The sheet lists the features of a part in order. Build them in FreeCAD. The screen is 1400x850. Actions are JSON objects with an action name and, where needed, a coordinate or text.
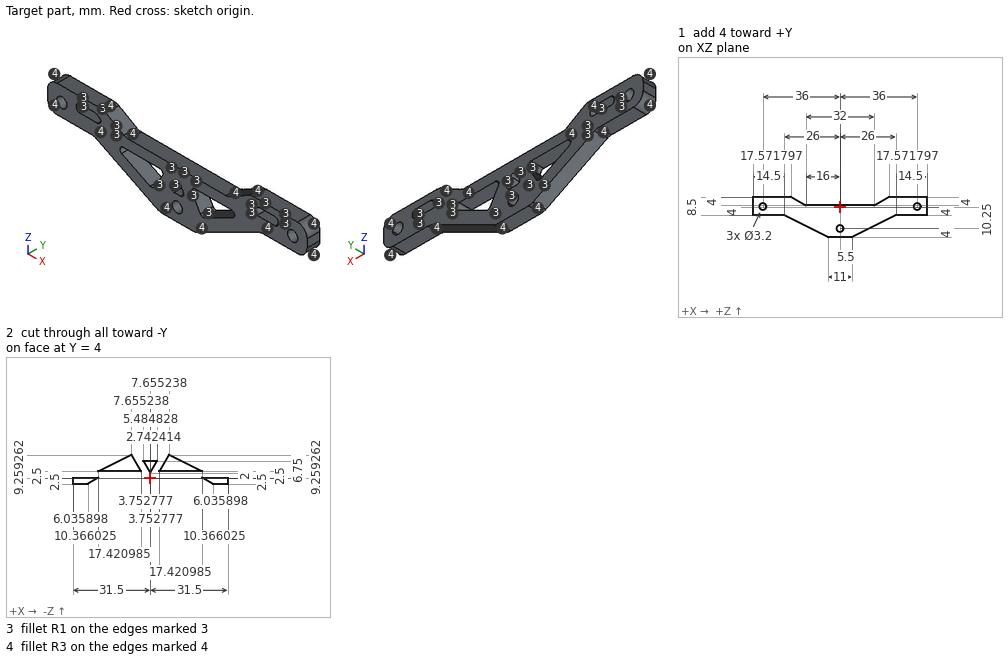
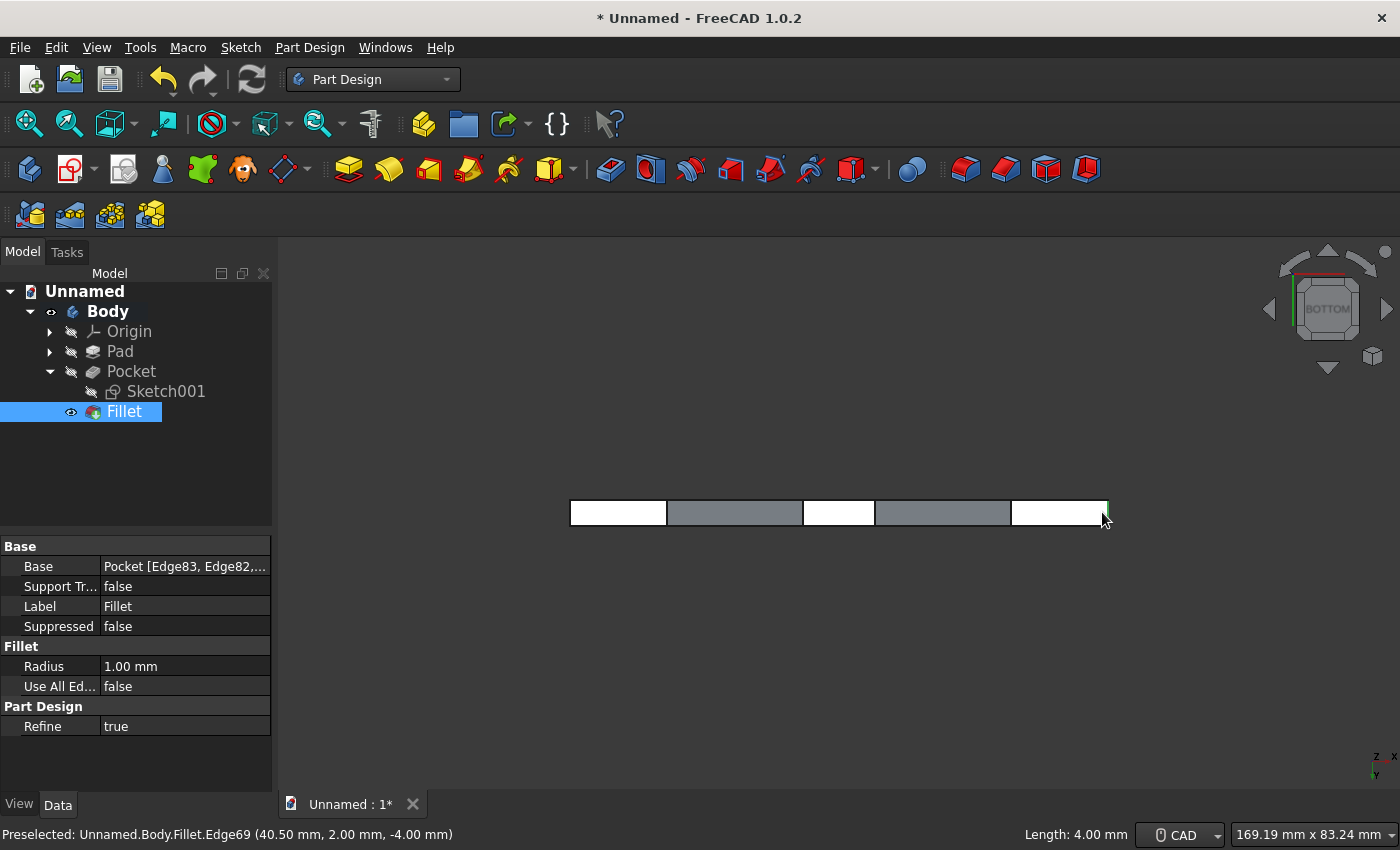
{"action": "left_click", "coordinate": [570, 512], "text": "ctrl"}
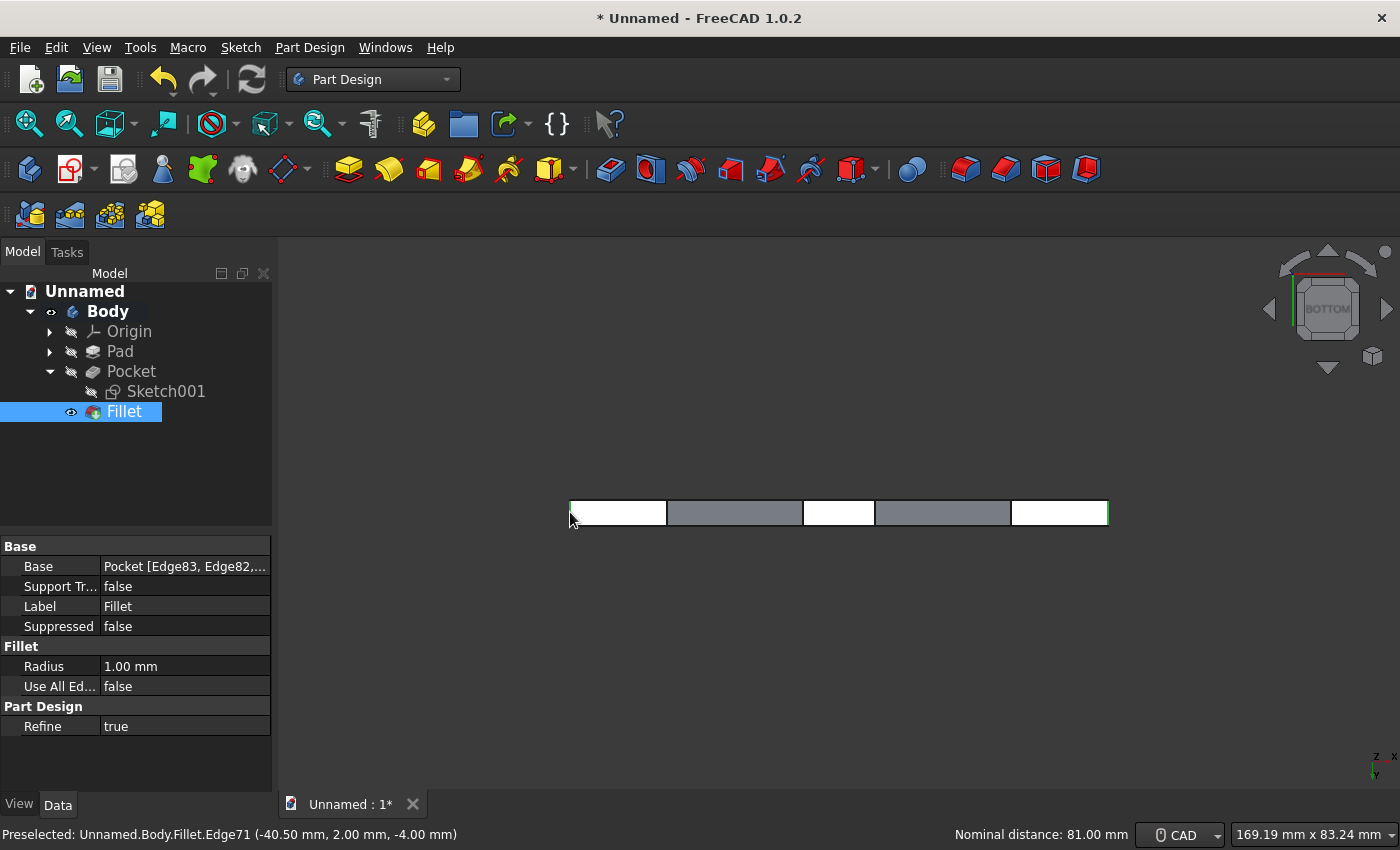
{"action": "left_click", "coordinate": [803, 512], "text": "ctrl"}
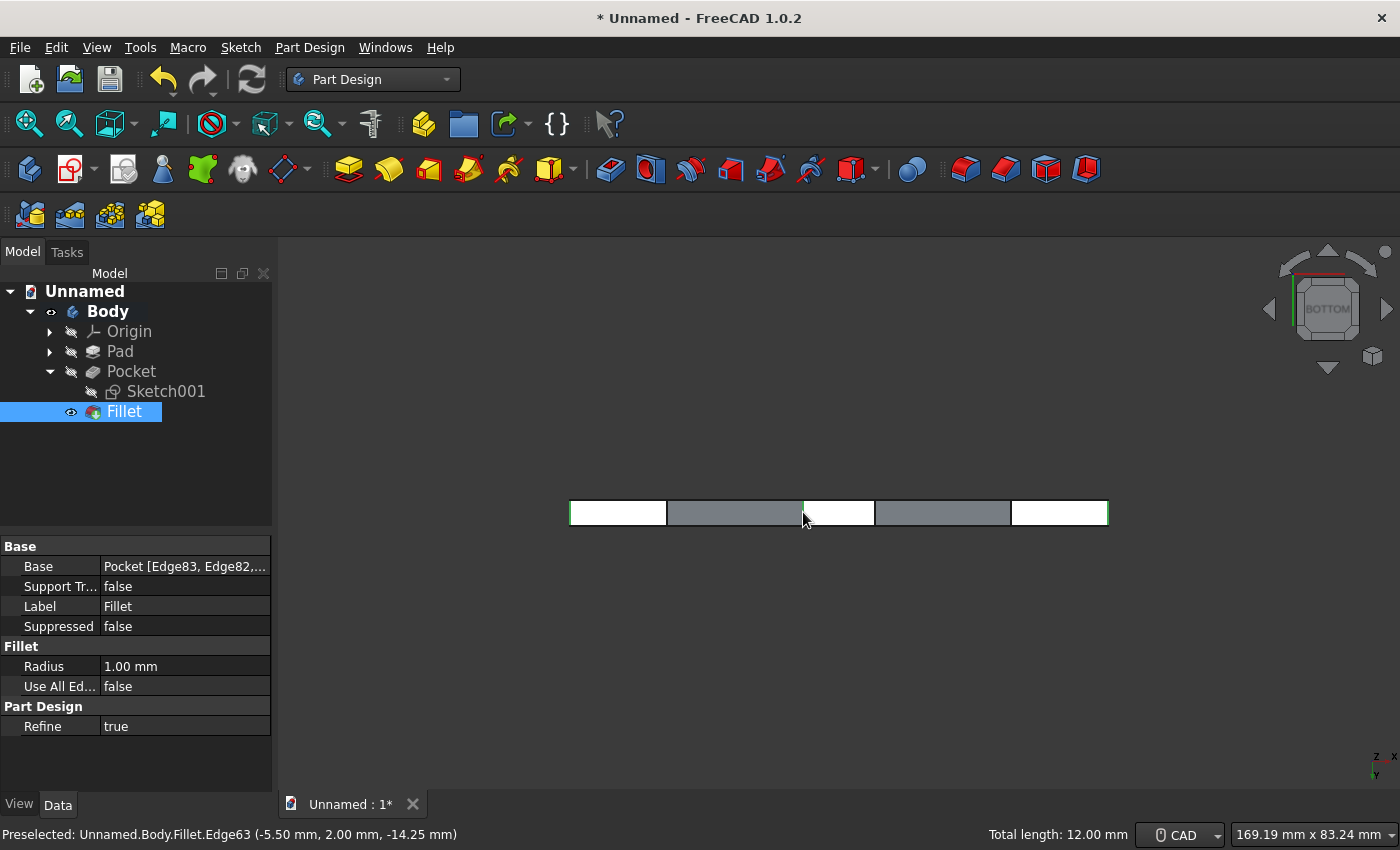
{"action": "left_click", "coordinate": [875, 512], "text": "ctrl"}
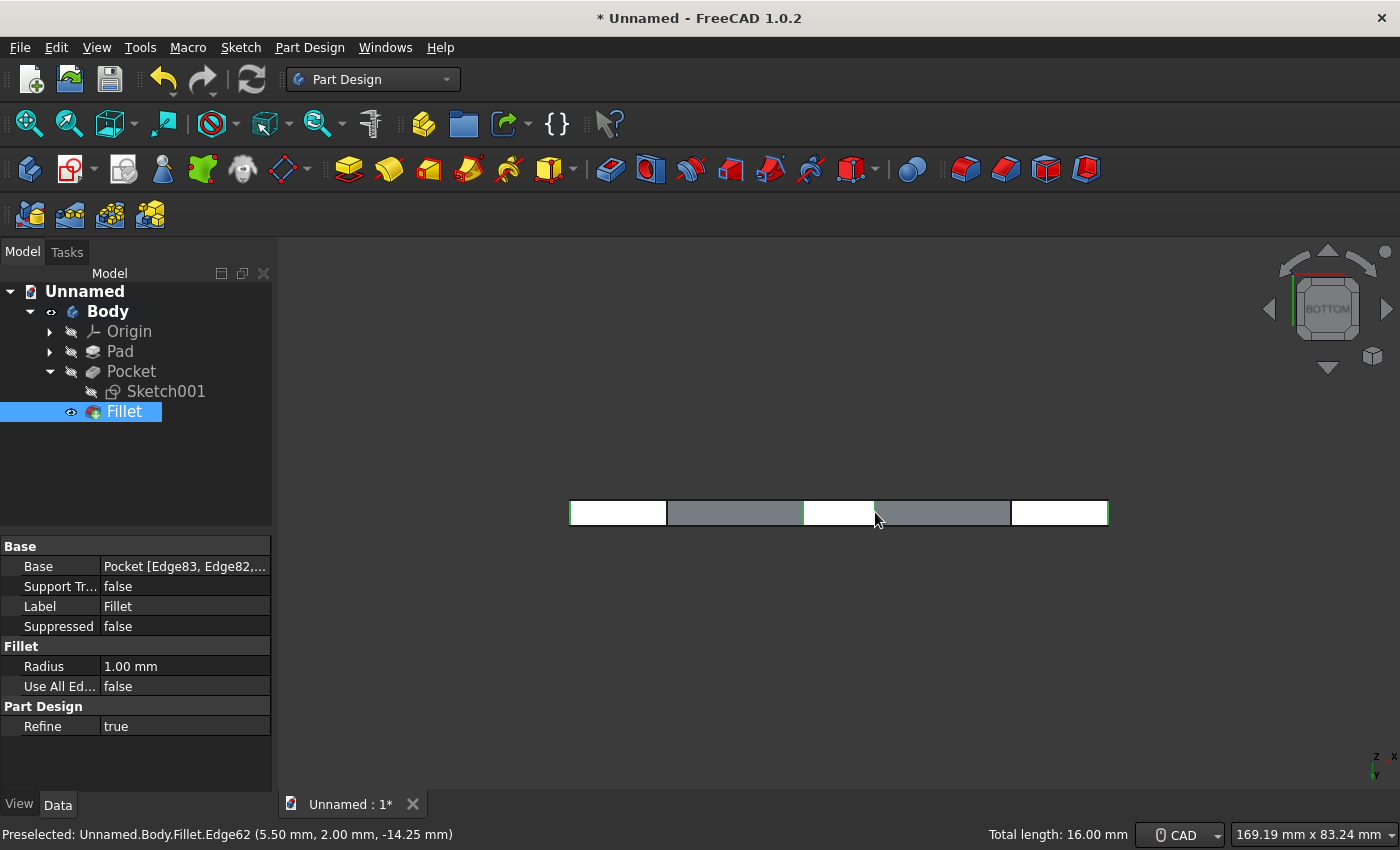
{"action": "key", "text": "0"}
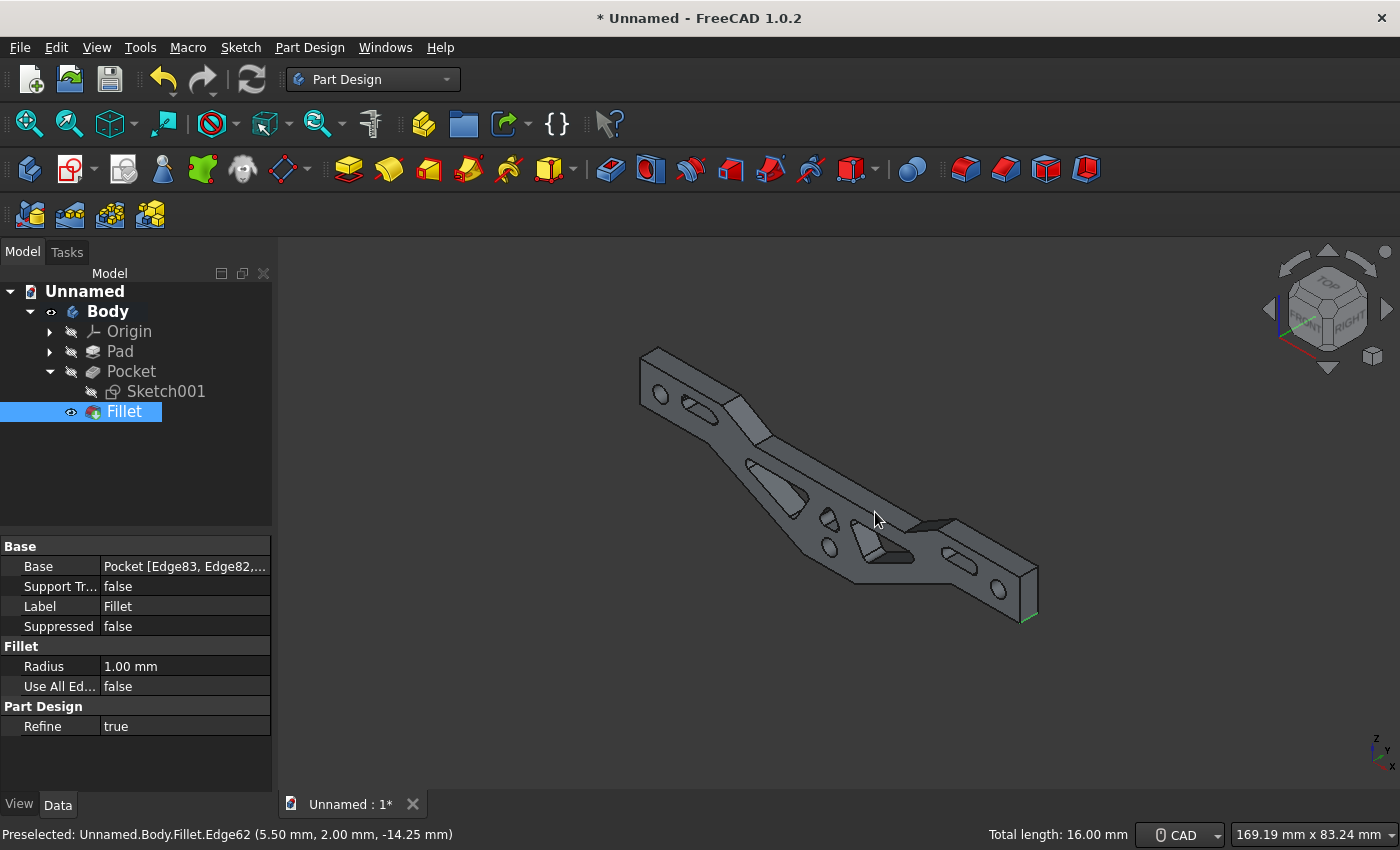
{"action": "left_click", "coordinate": [1029, 571], "text": "ctrl"}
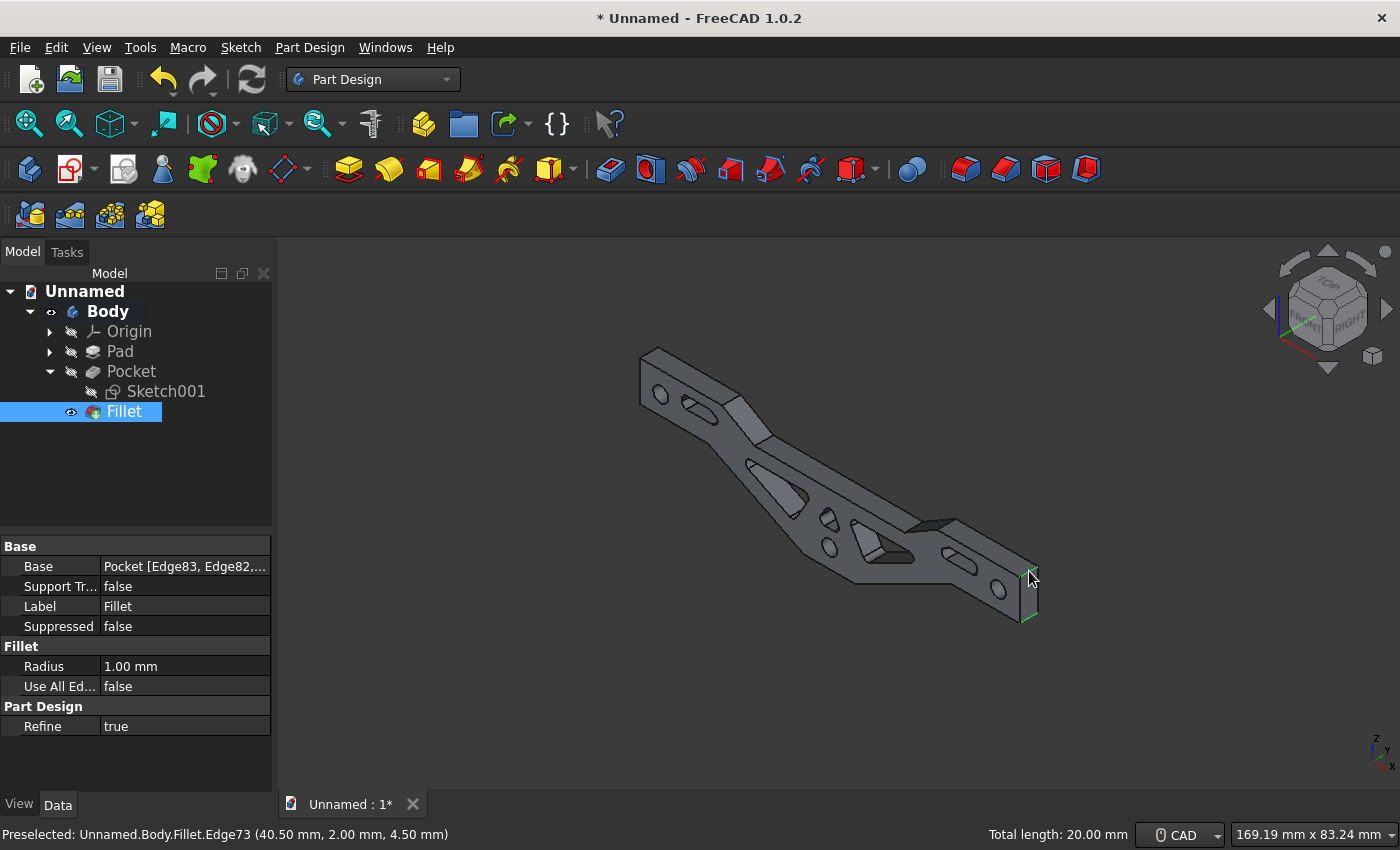
{"action": "key", "text": "2"}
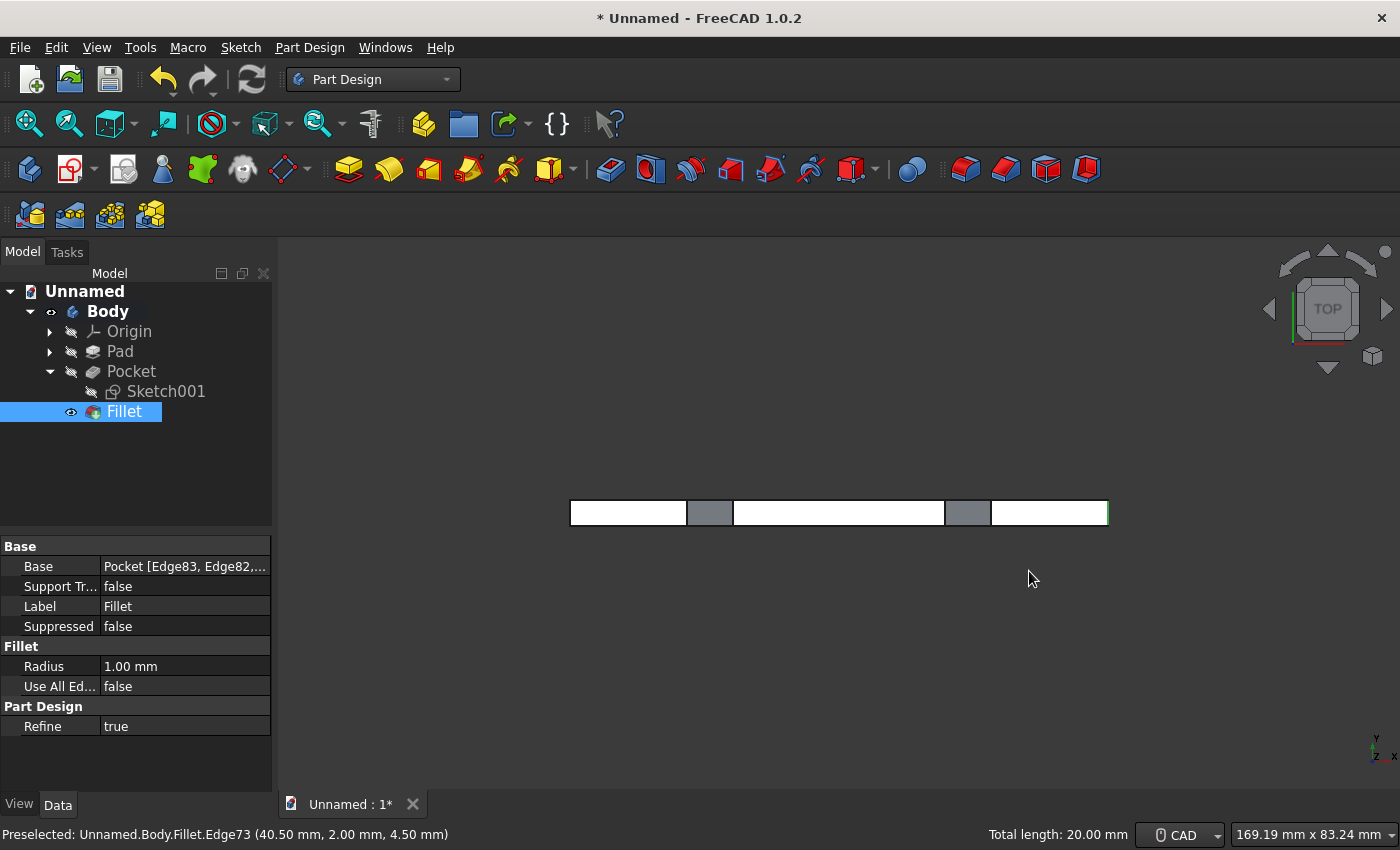
{"action": "left_click", "coordinate": [991, 512], "text": "ctrl"}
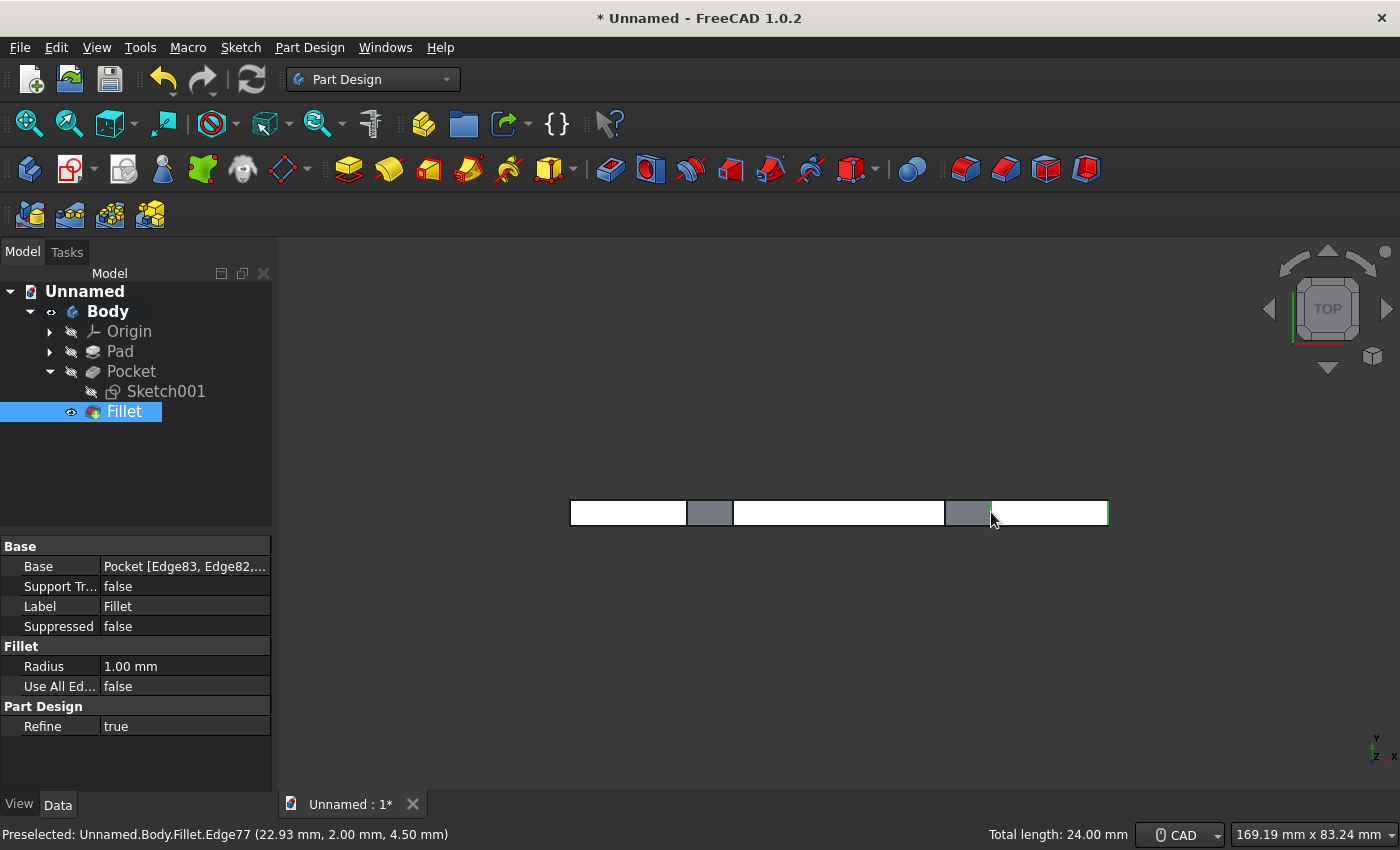
{"action": "left_click", "coordinate": [687, 512], "text": "ctrl"}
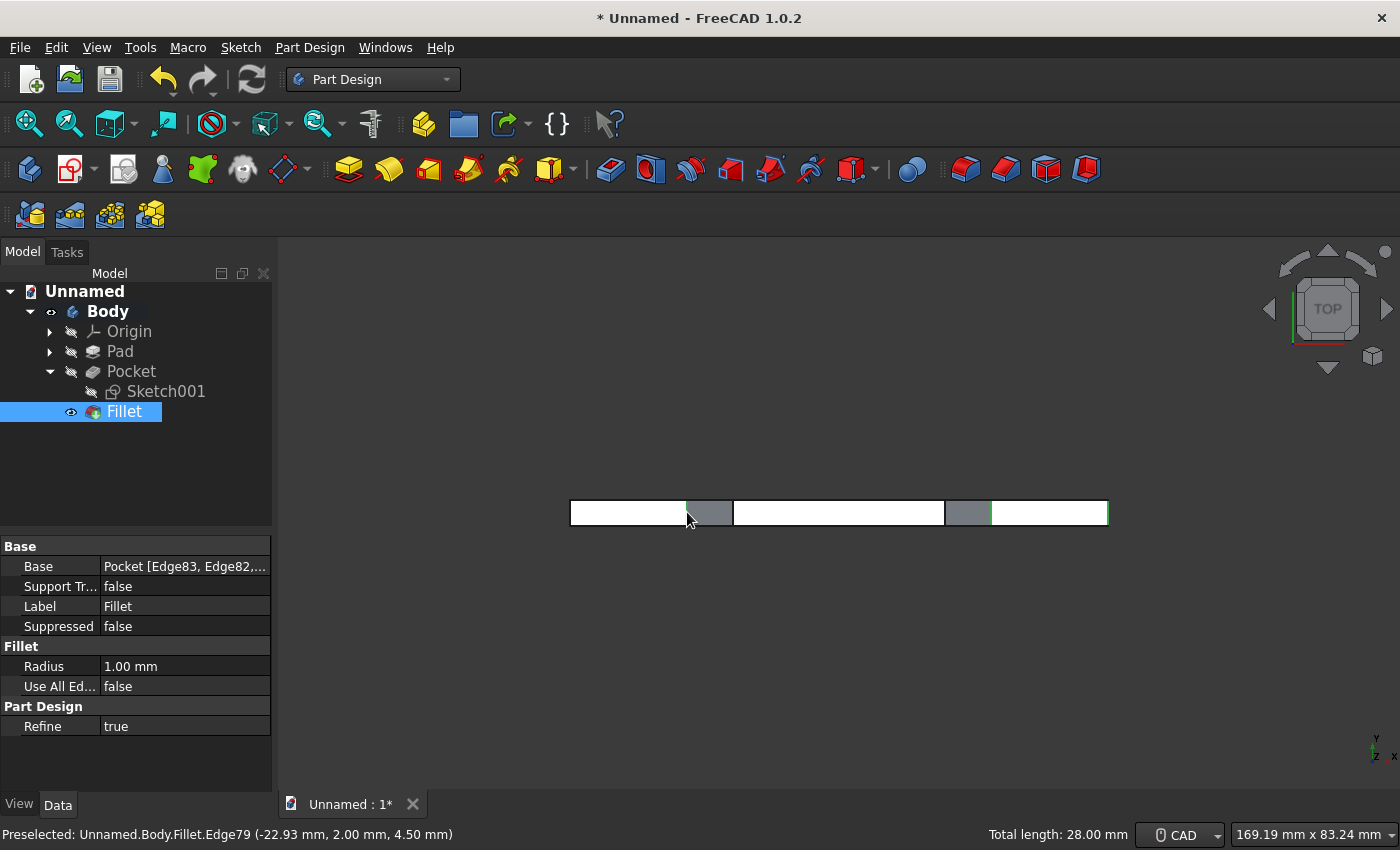
{"action": "left_click", "coordinate": [570, 512], "text": "ctrl"}